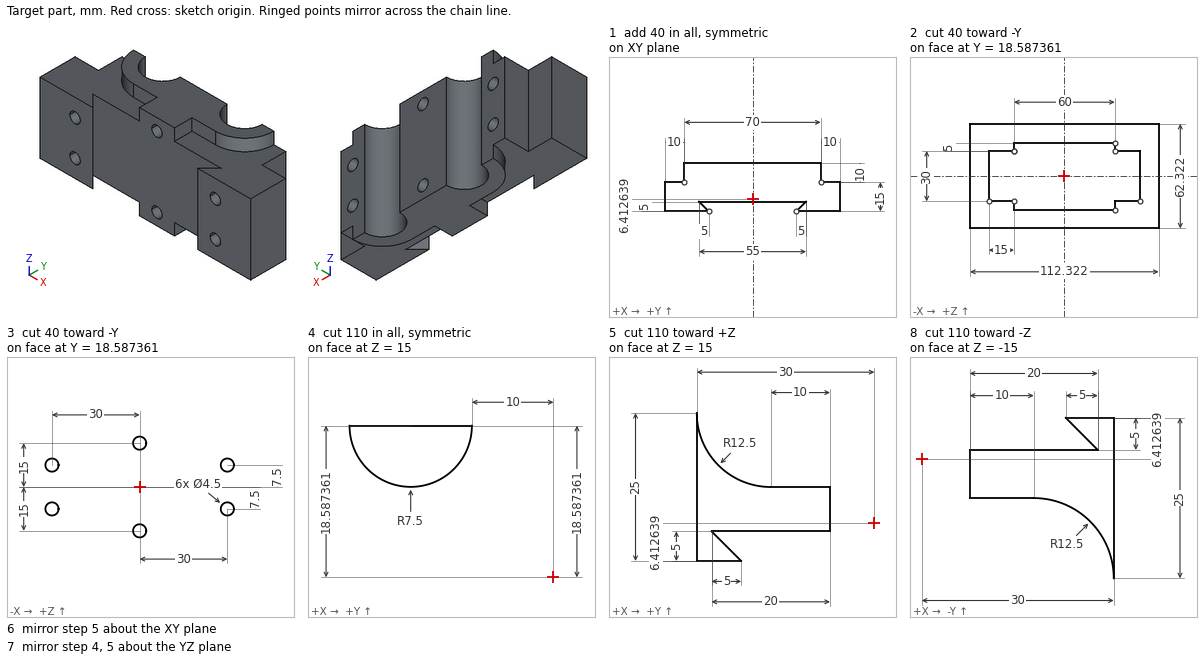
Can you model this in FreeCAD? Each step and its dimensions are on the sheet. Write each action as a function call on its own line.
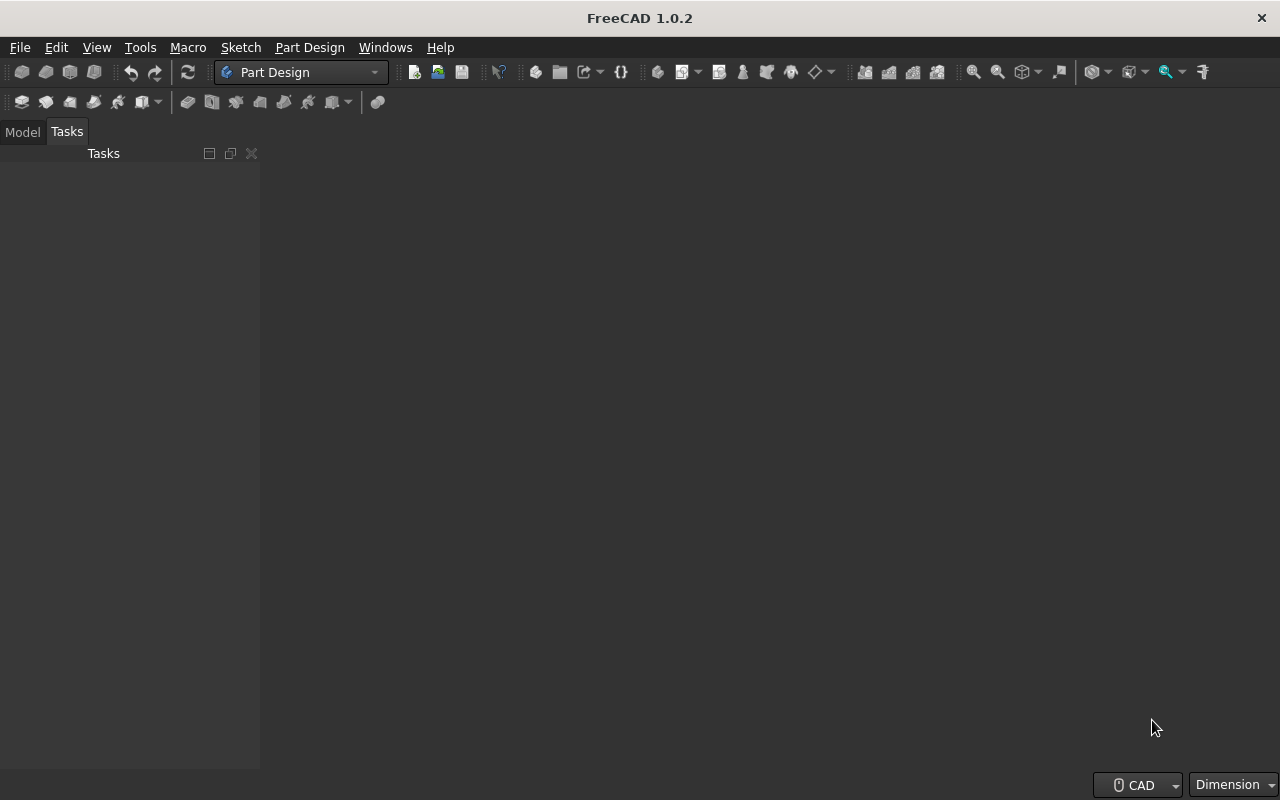
key(ctrl+n)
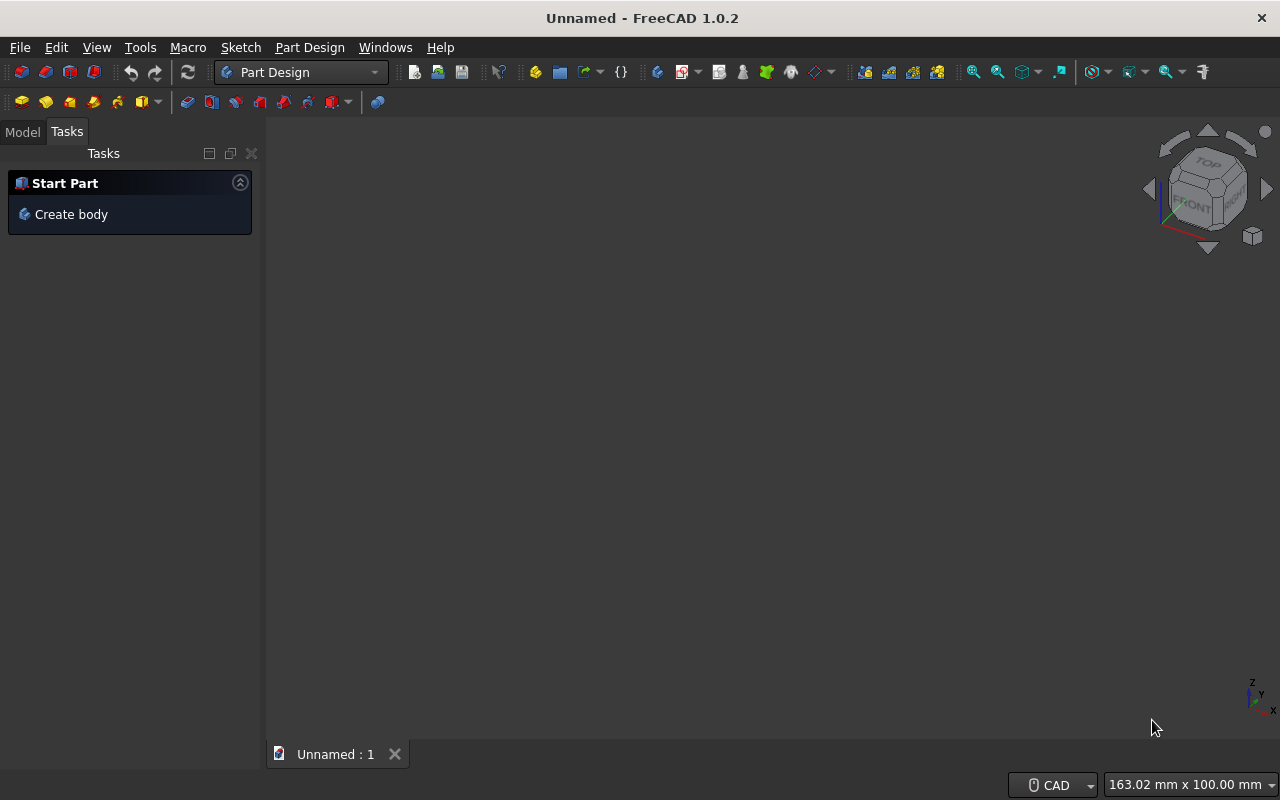
click(682, 72)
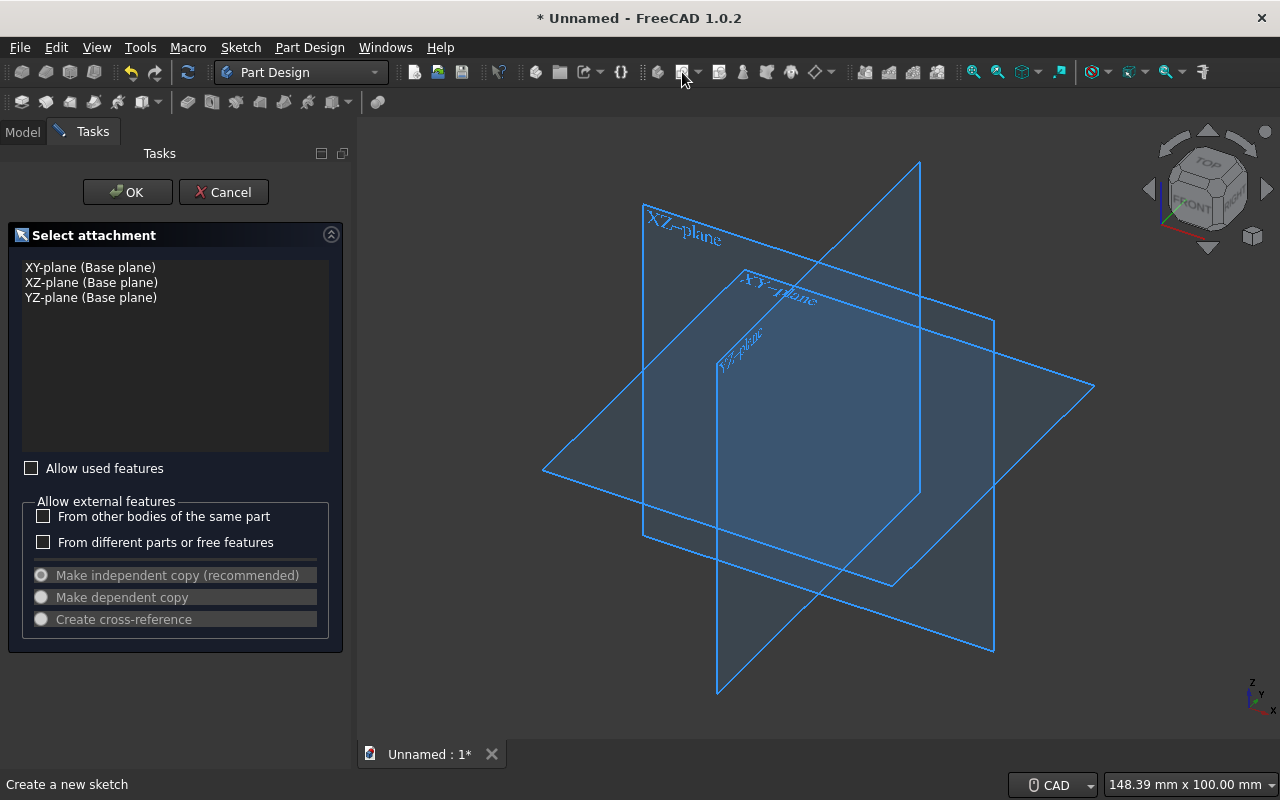
click(82, 268)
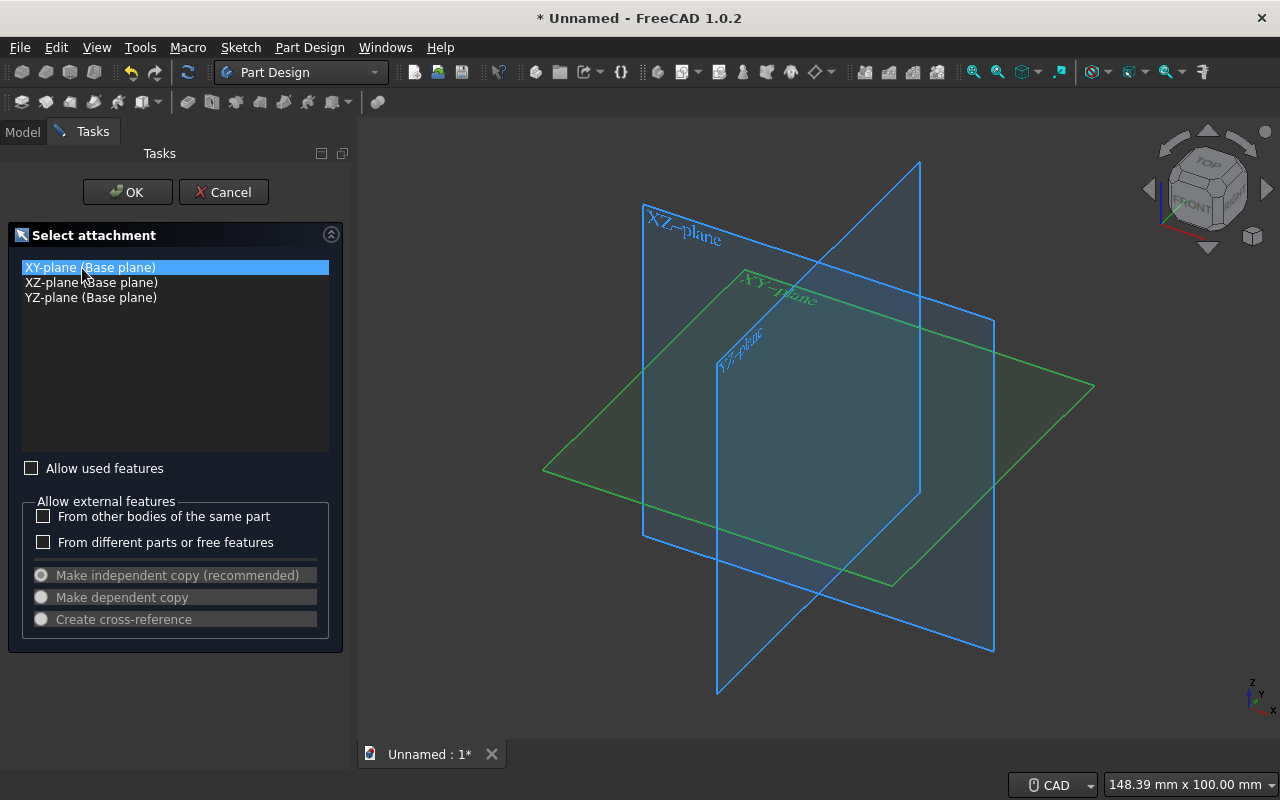
click(128, 192)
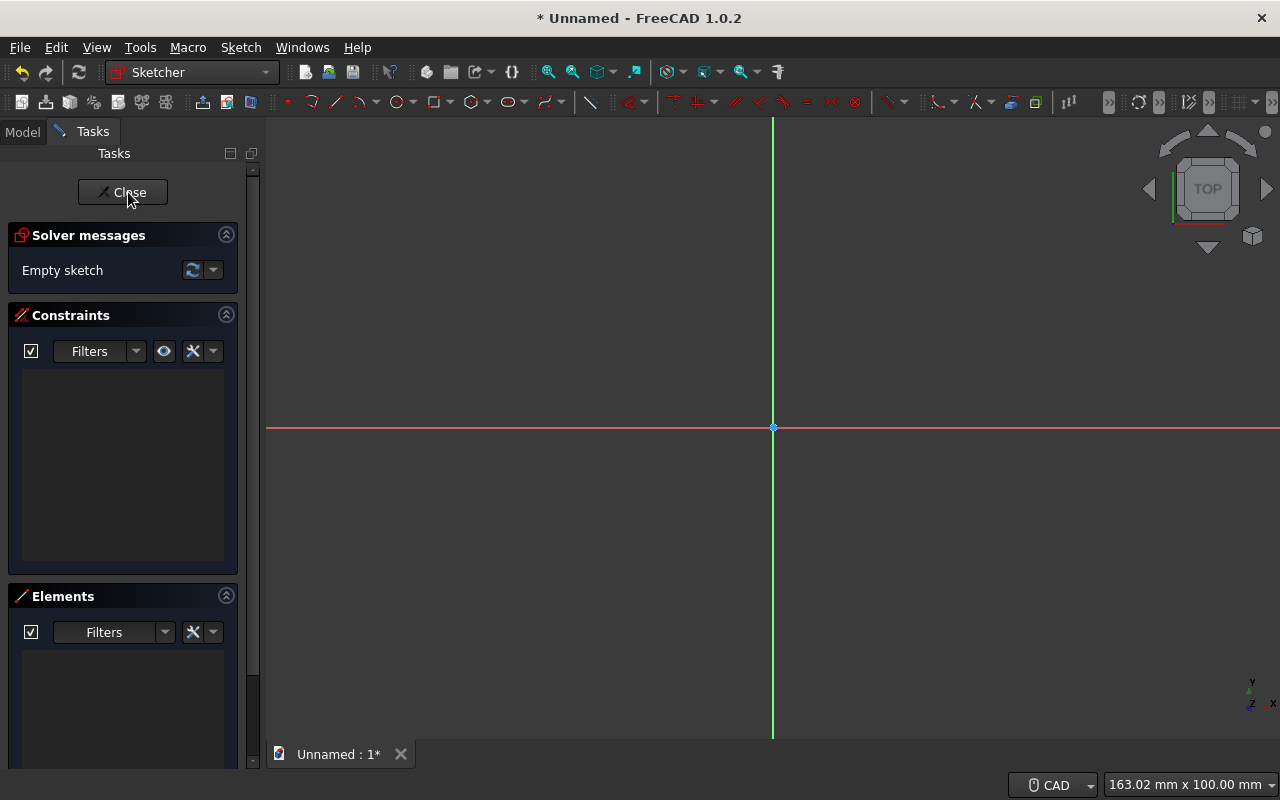
key(g)
key(m)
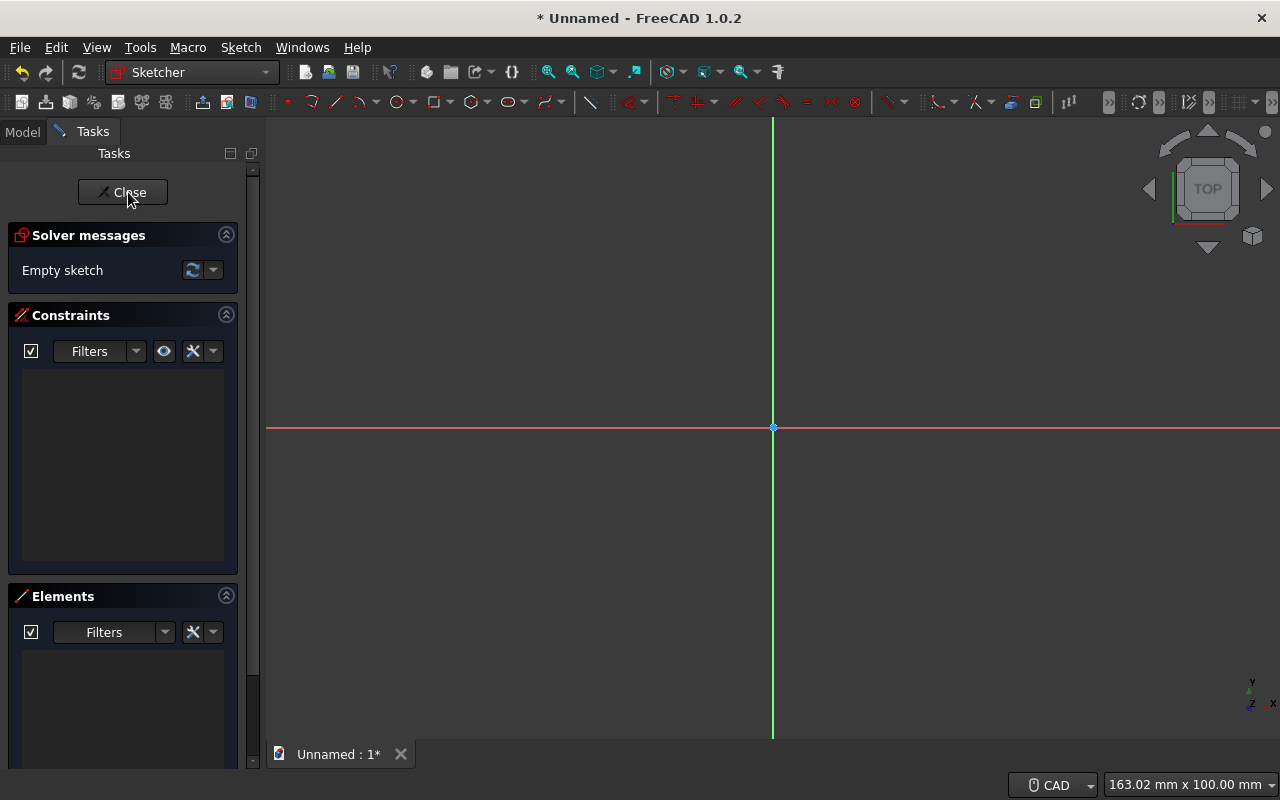
click(633, 468)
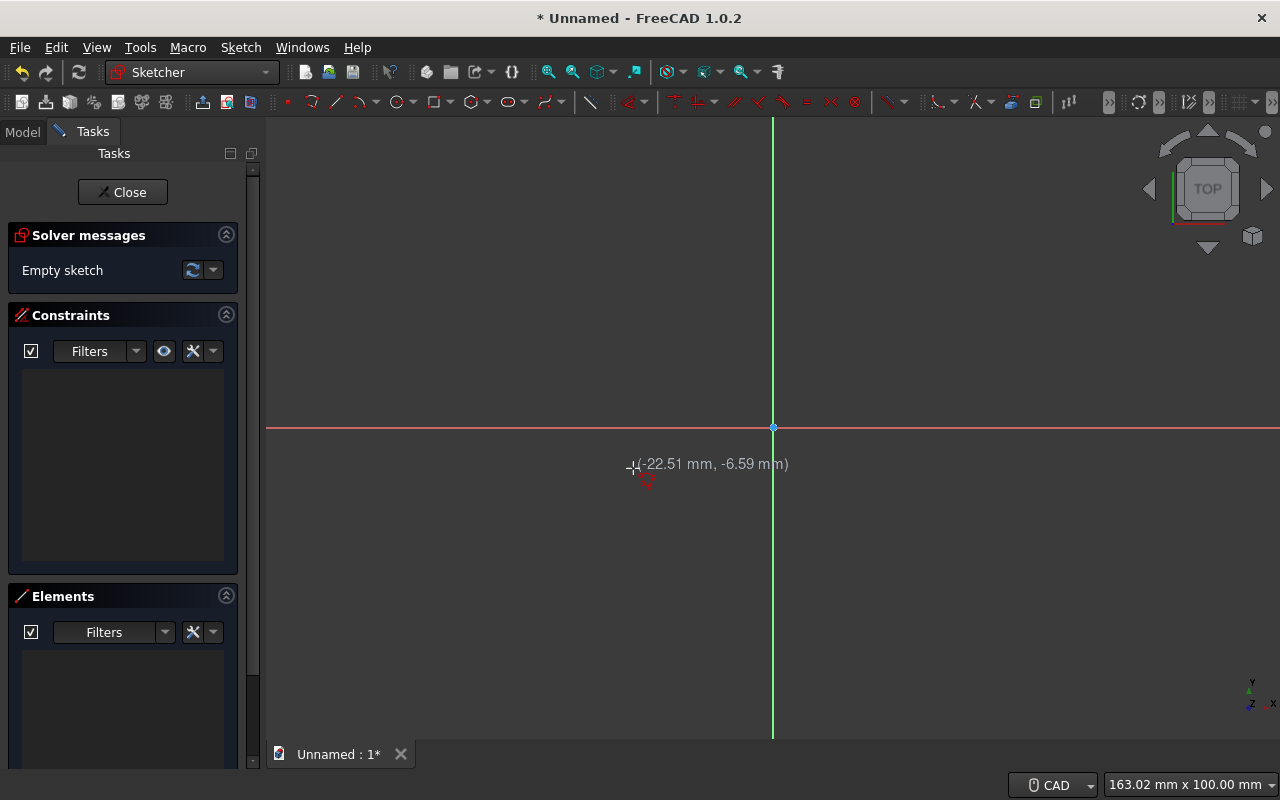
scroll(602, 437, up, 3)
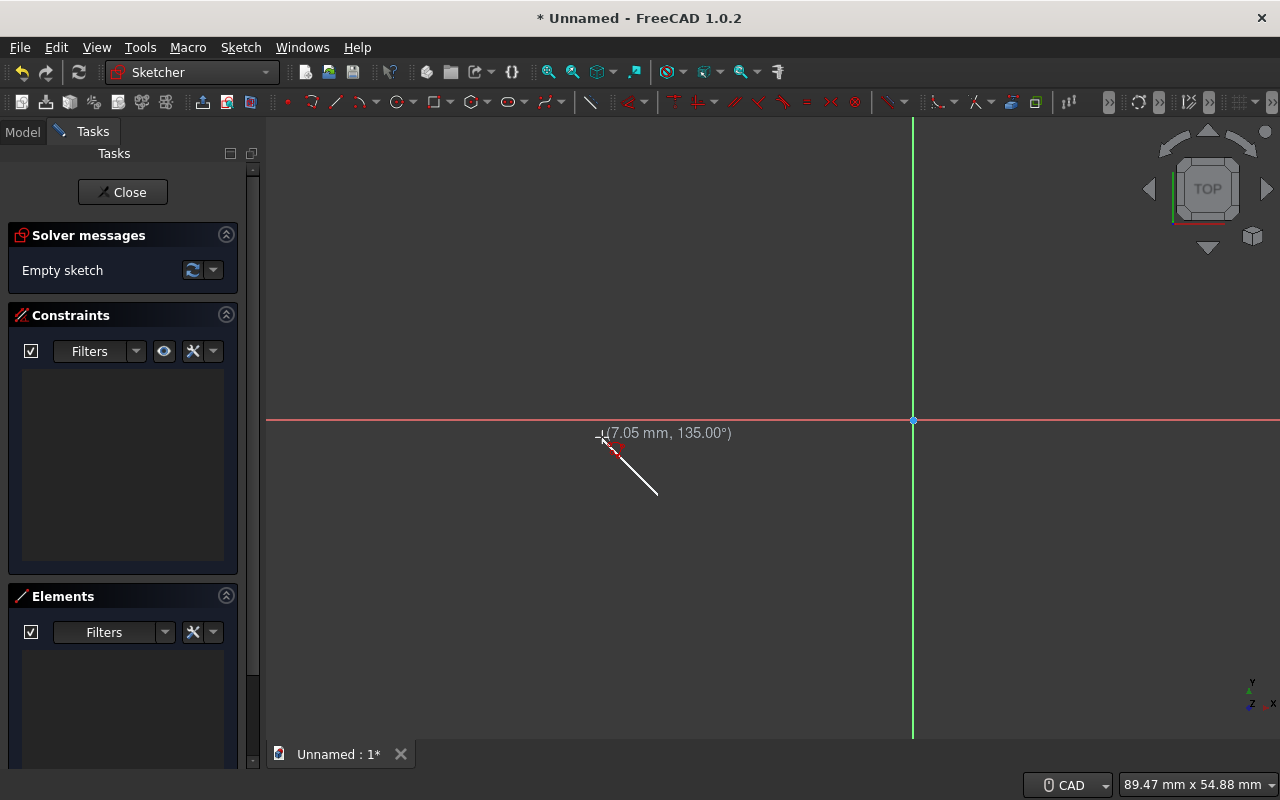
click(602, 436)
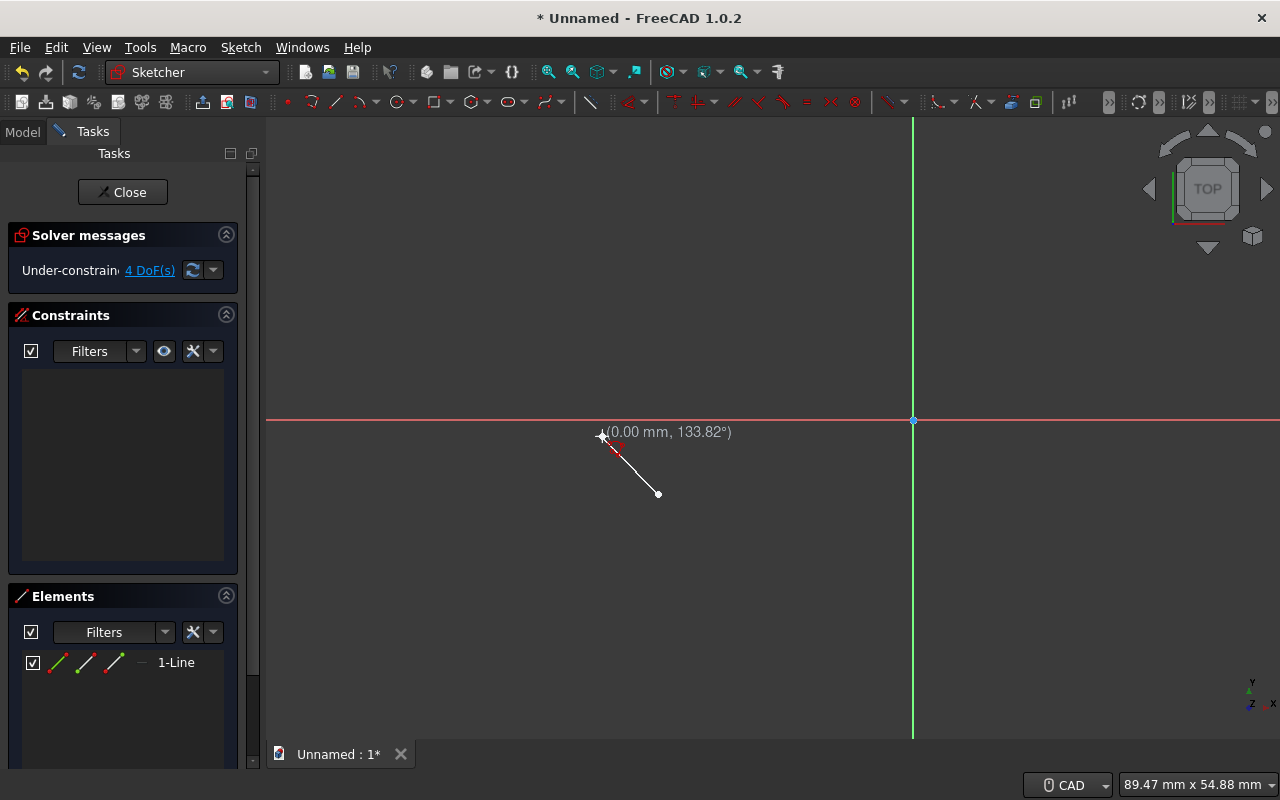
scroll(451, 521, down, 3)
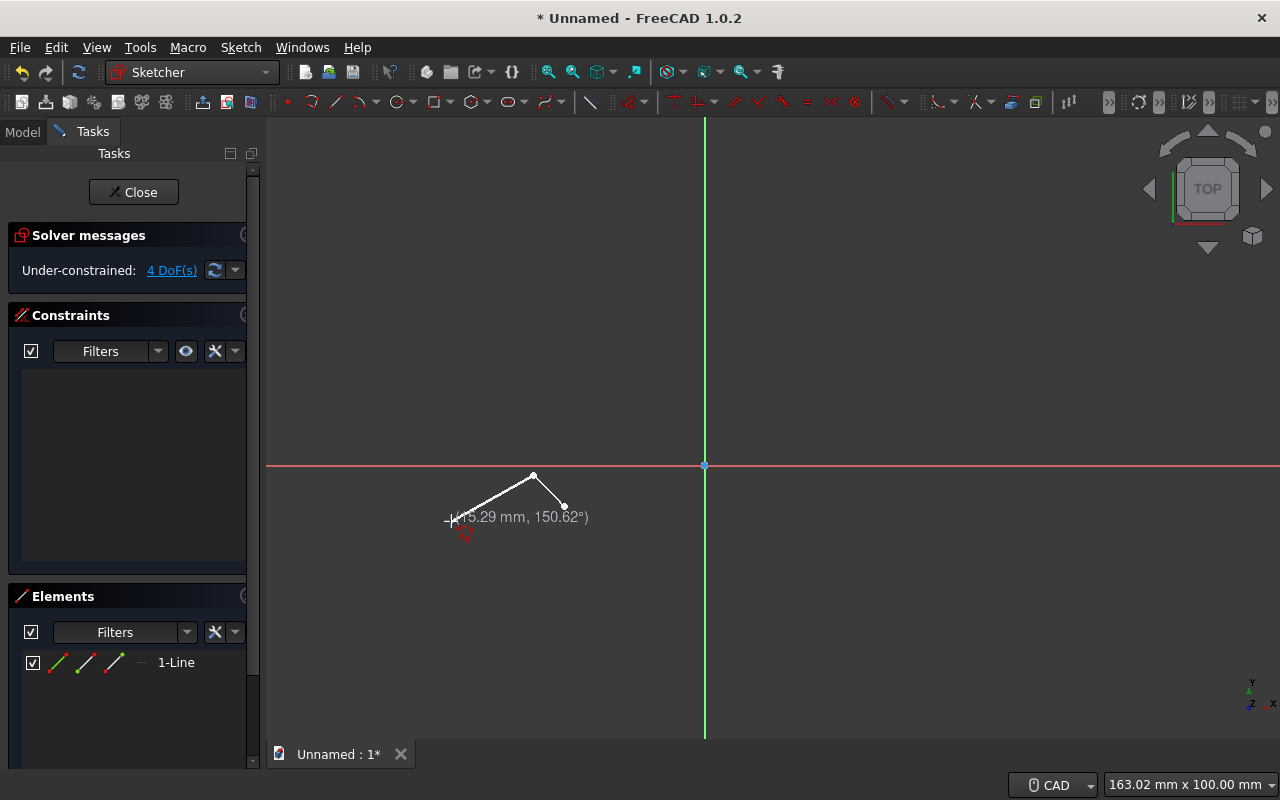
scroll(876, 475, up, 3)